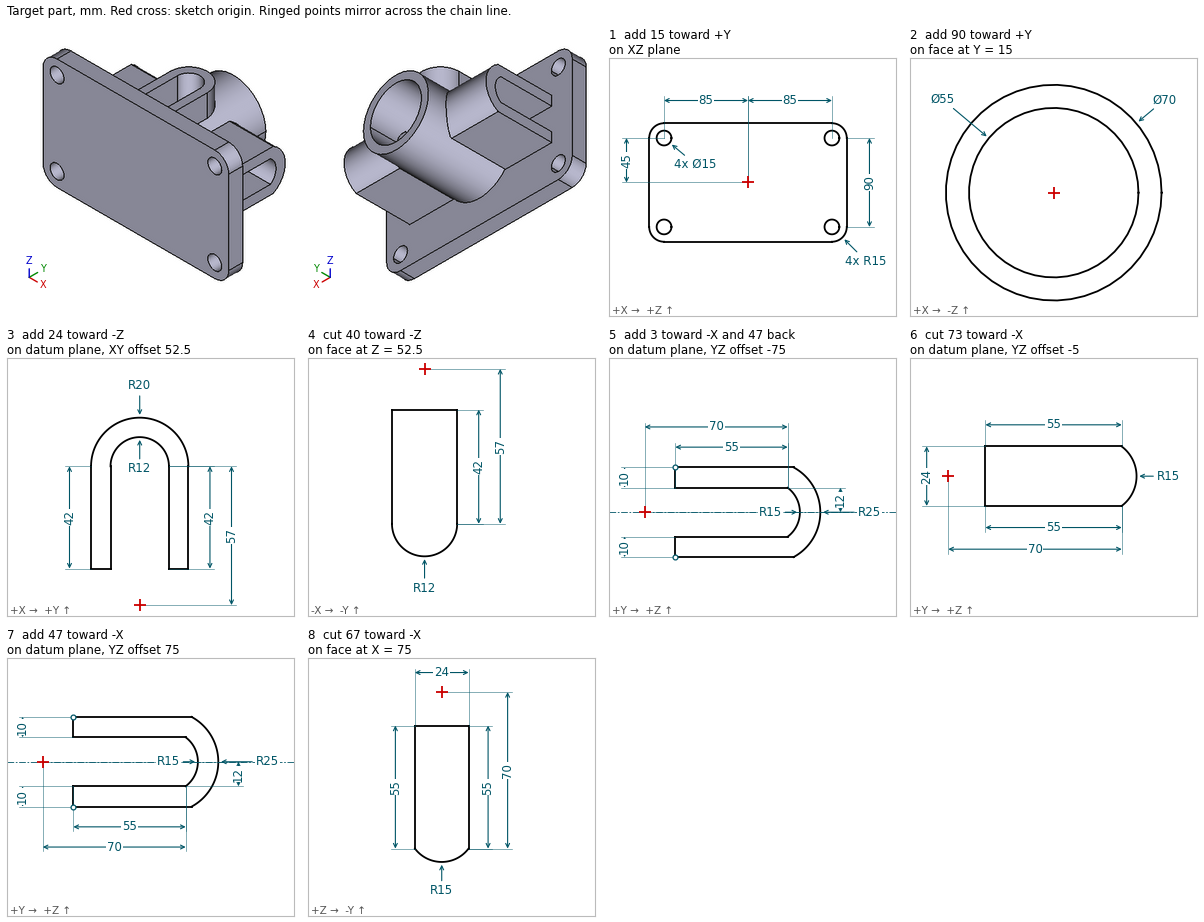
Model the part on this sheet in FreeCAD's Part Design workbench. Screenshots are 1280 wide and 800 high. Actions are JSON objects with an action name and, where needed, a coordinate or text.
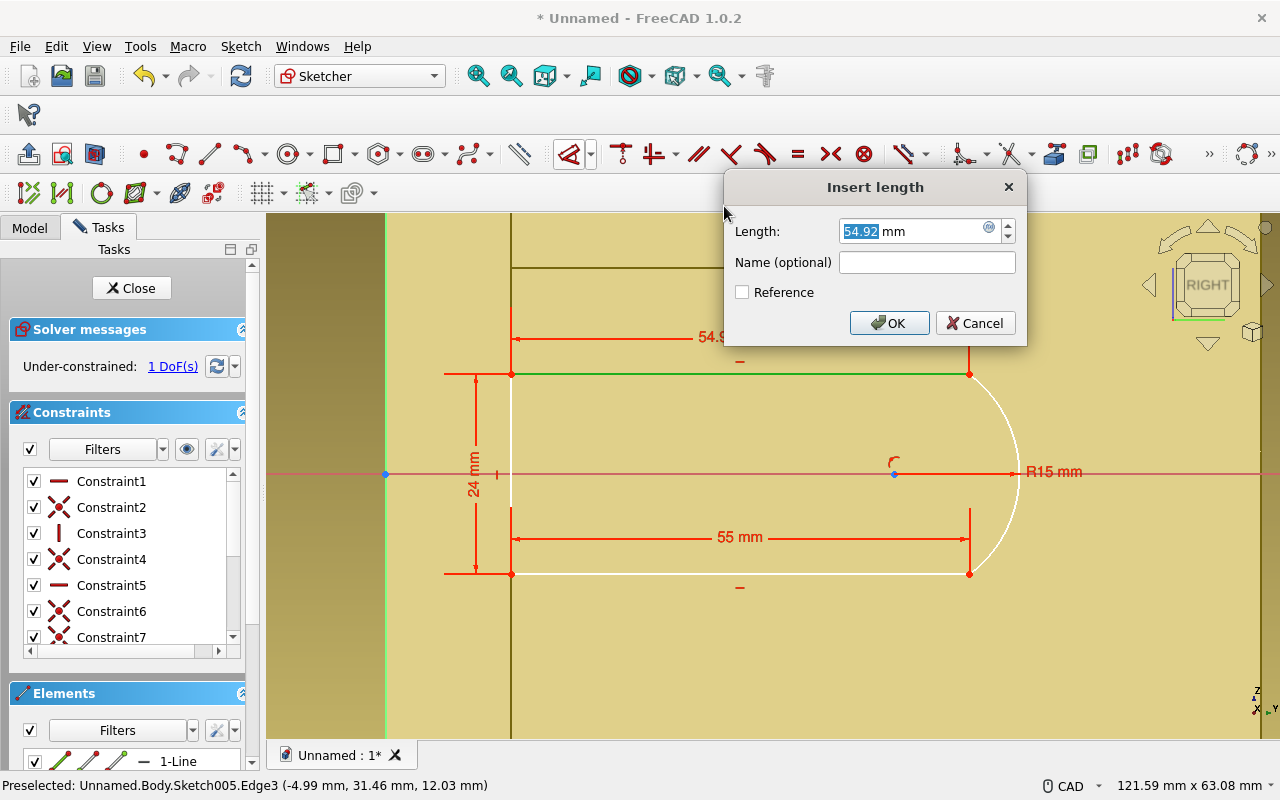
{"action": "type", "text": "55"}
{"action": "key", "text": "Return"}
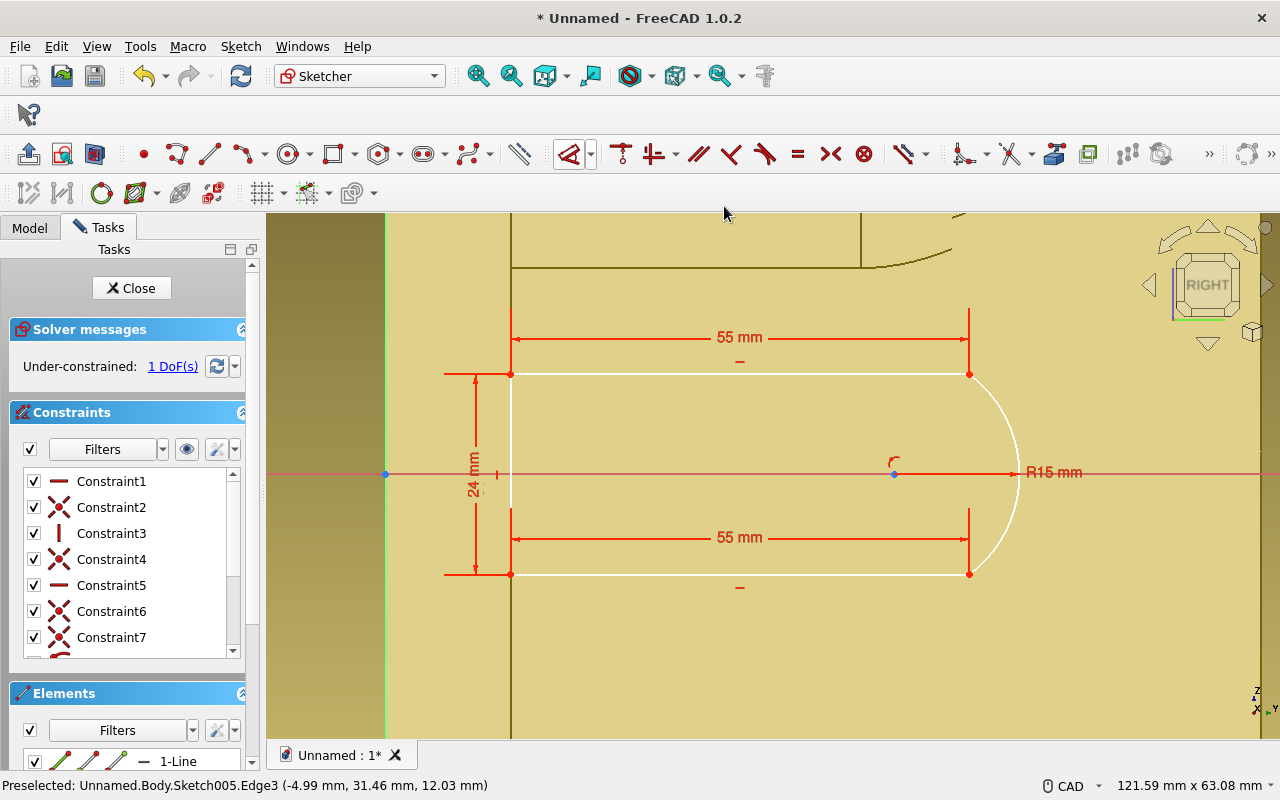
{"action": "left_click", "coordinate": [969, 575]}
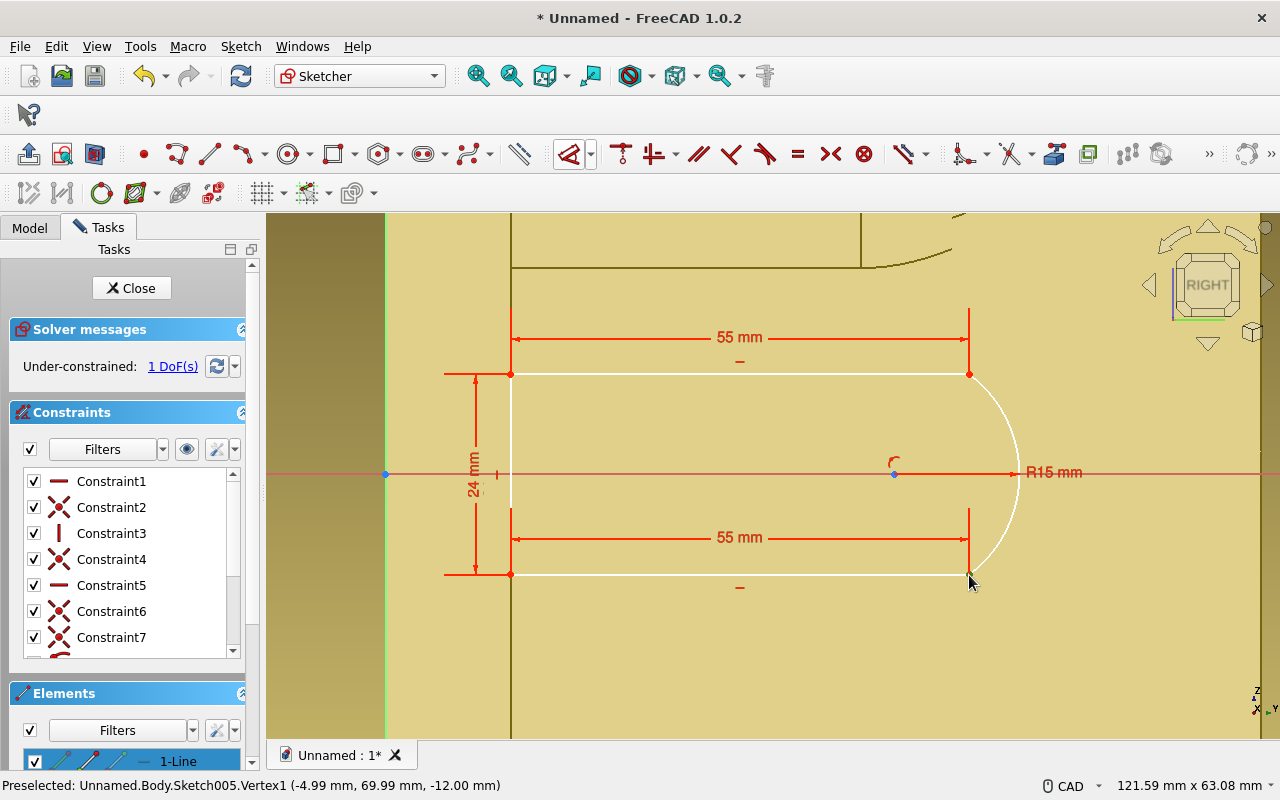
{"action": "key", "text": "l"}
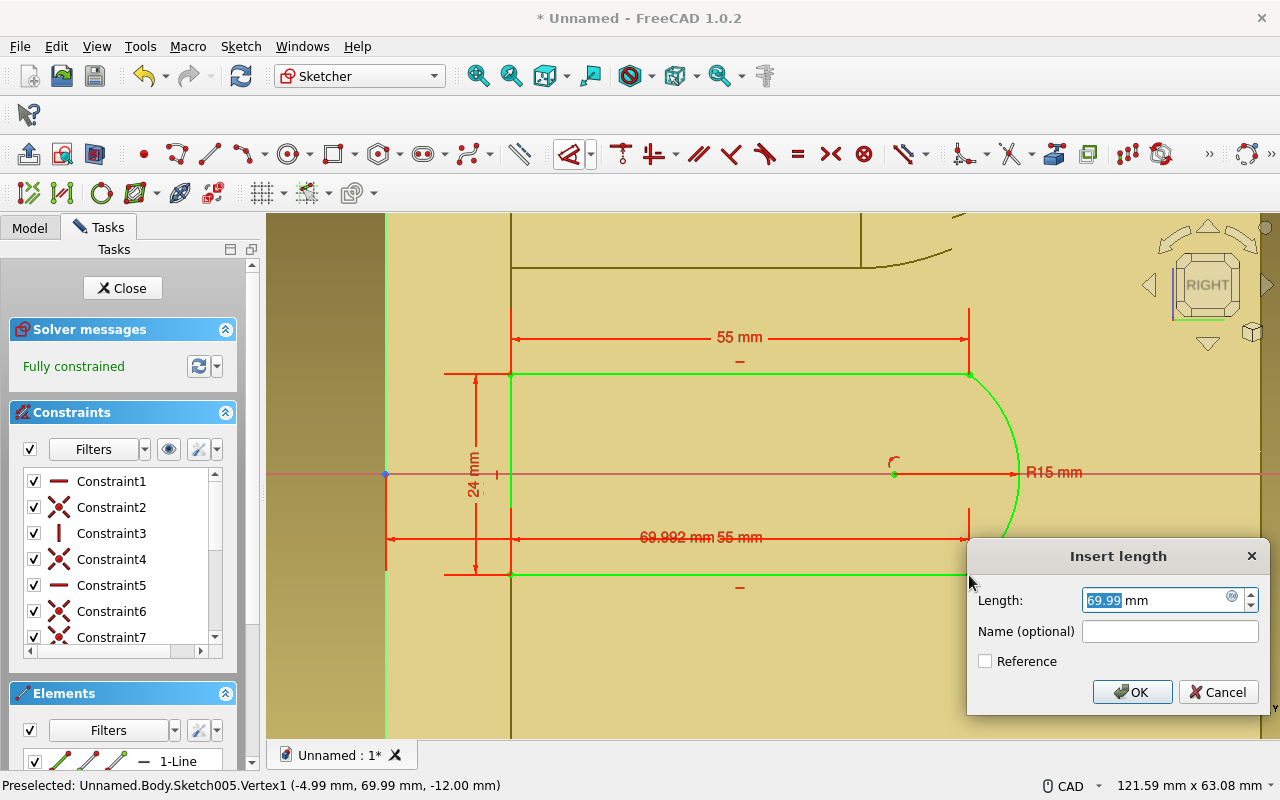
{"action": "type", "text": "70"}
{"action": "key", "text": "Return"}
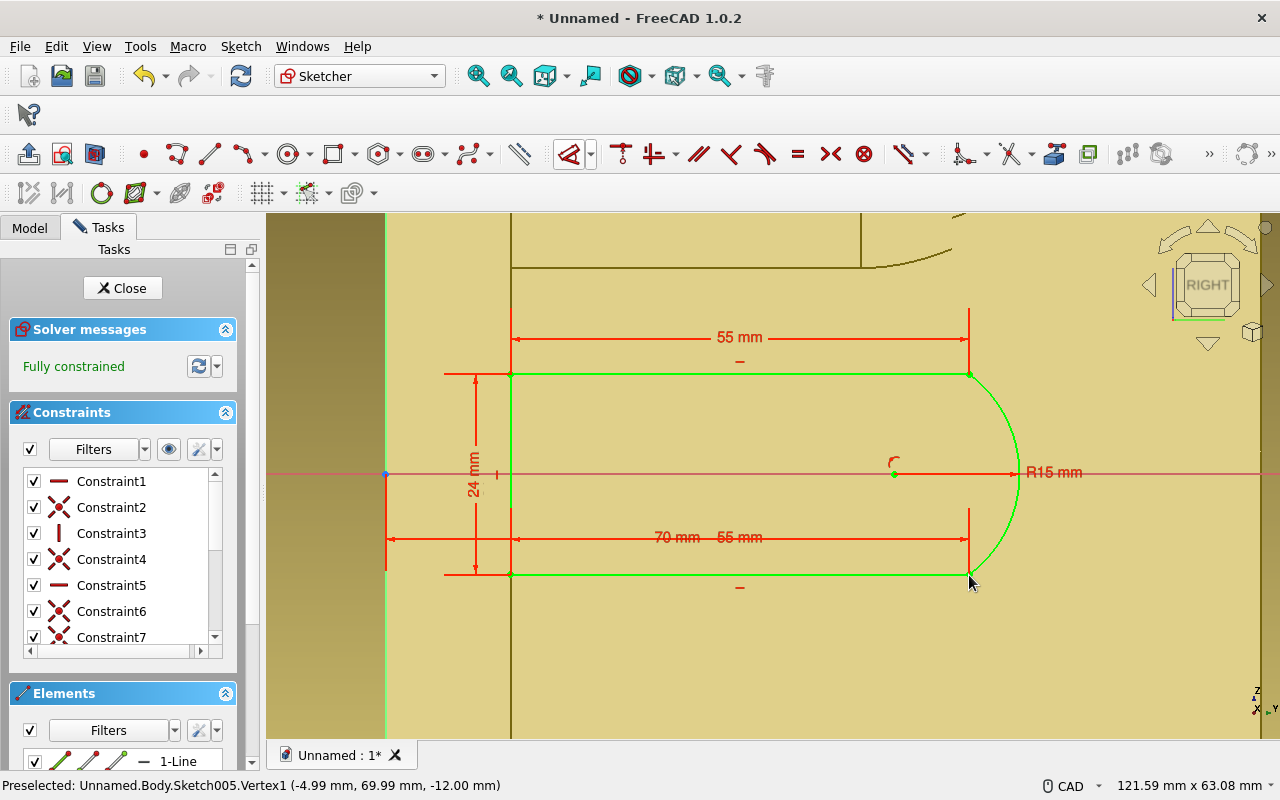
{"action": "left_click", "coordinate": [123, 288]}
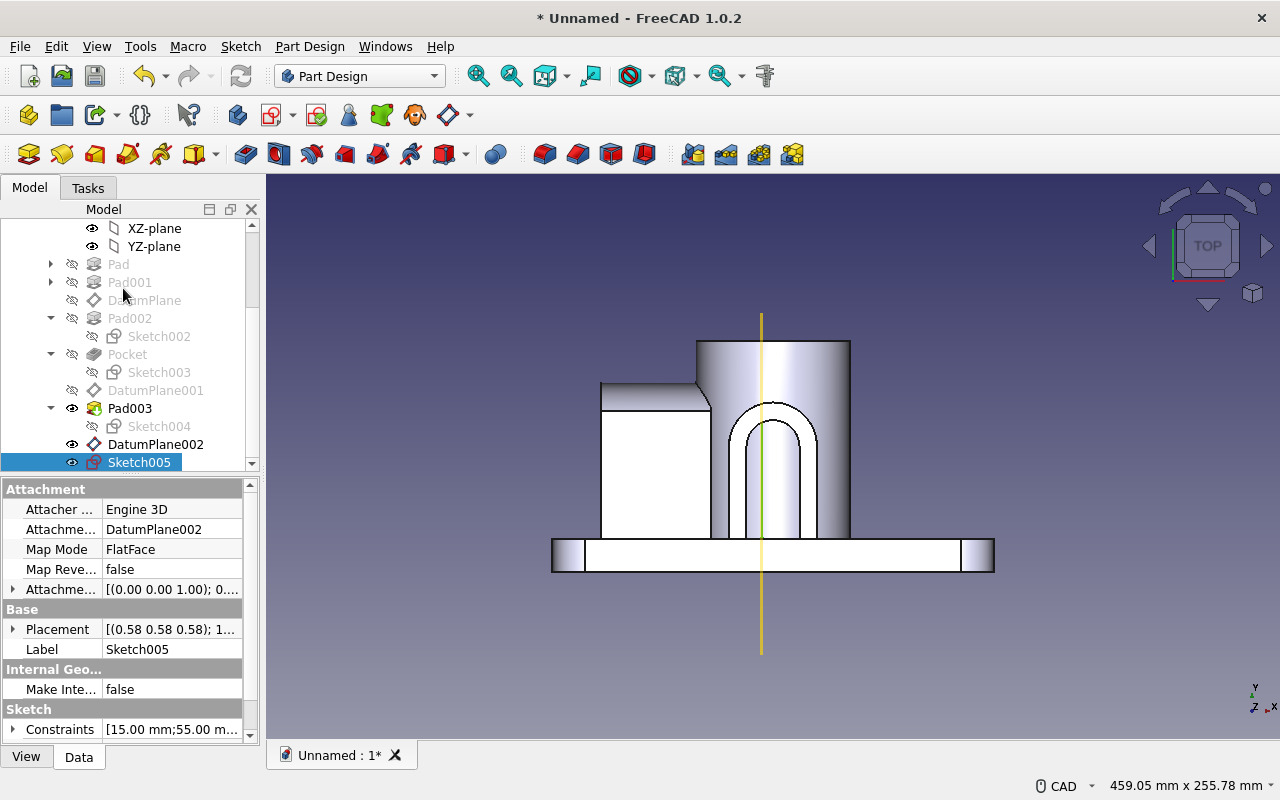
{"action": "left_click", "coordinate": [246, 154]}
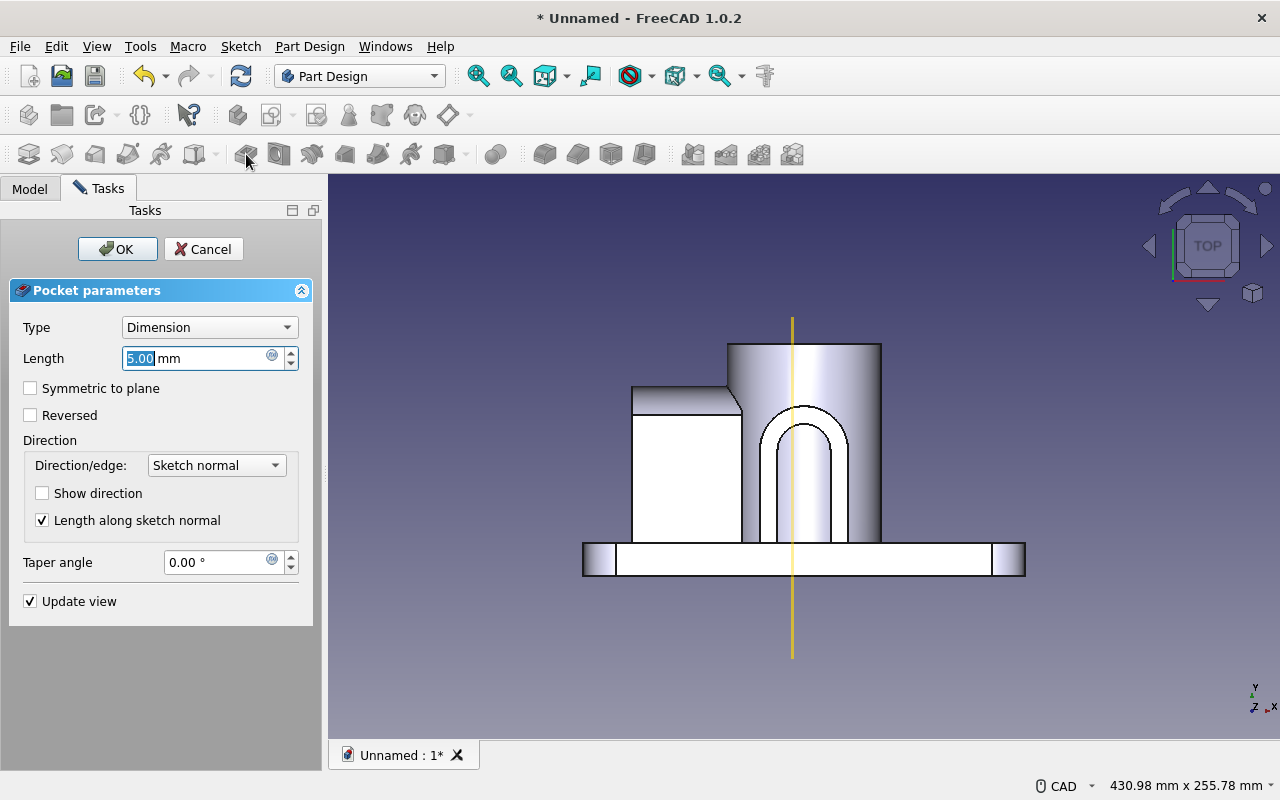
{"action": "type", "text": "73"}
{"action": "key", "text": "Tab"}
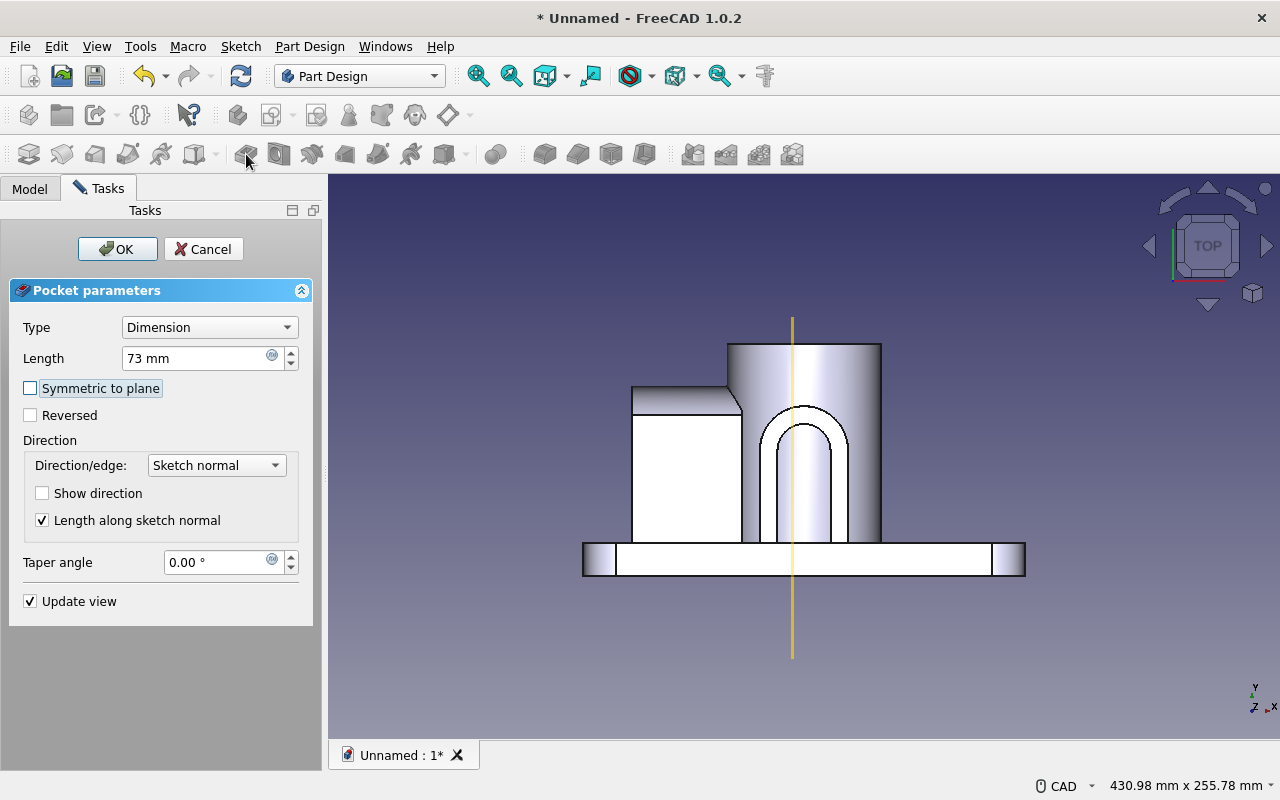
{"action": "left_click", "coordinate": [118, 249]}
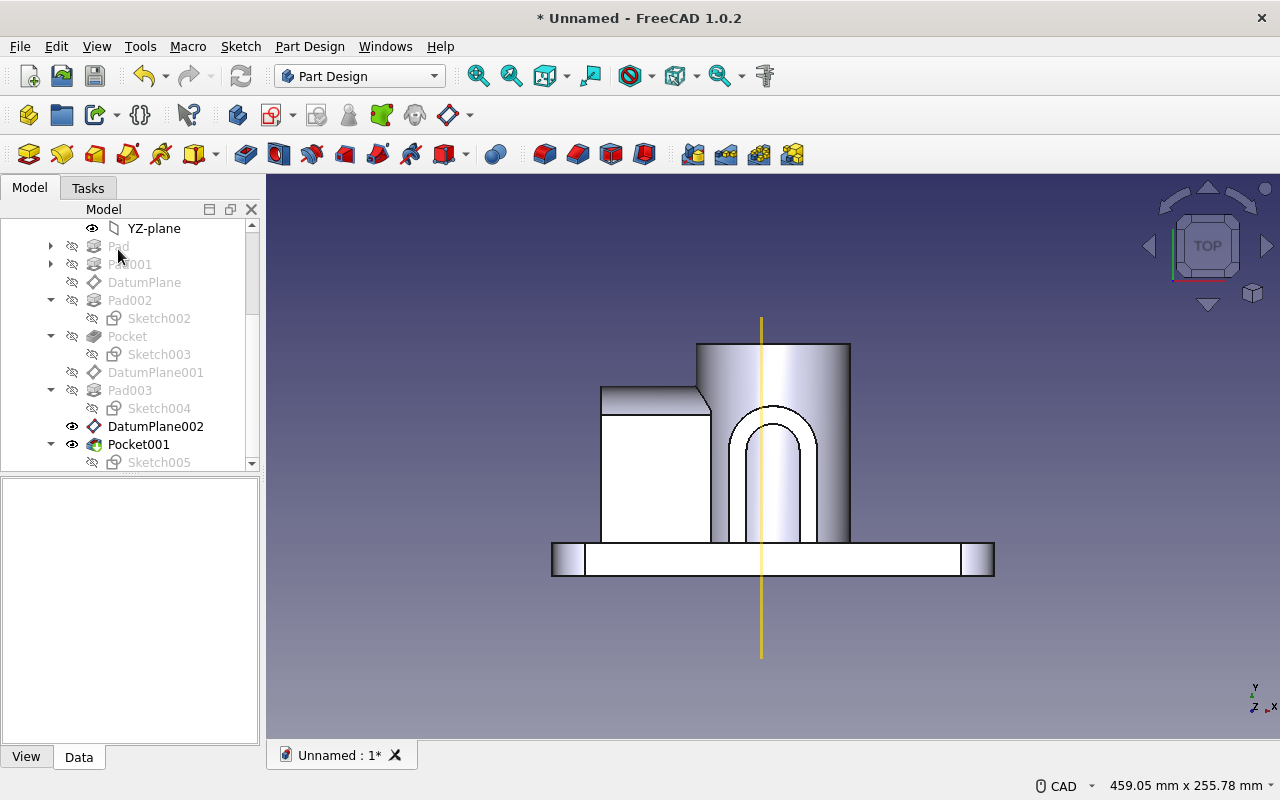
{"action": "left_click", "coordinate": [117, 426]}
{"action": "key", "text": "space"}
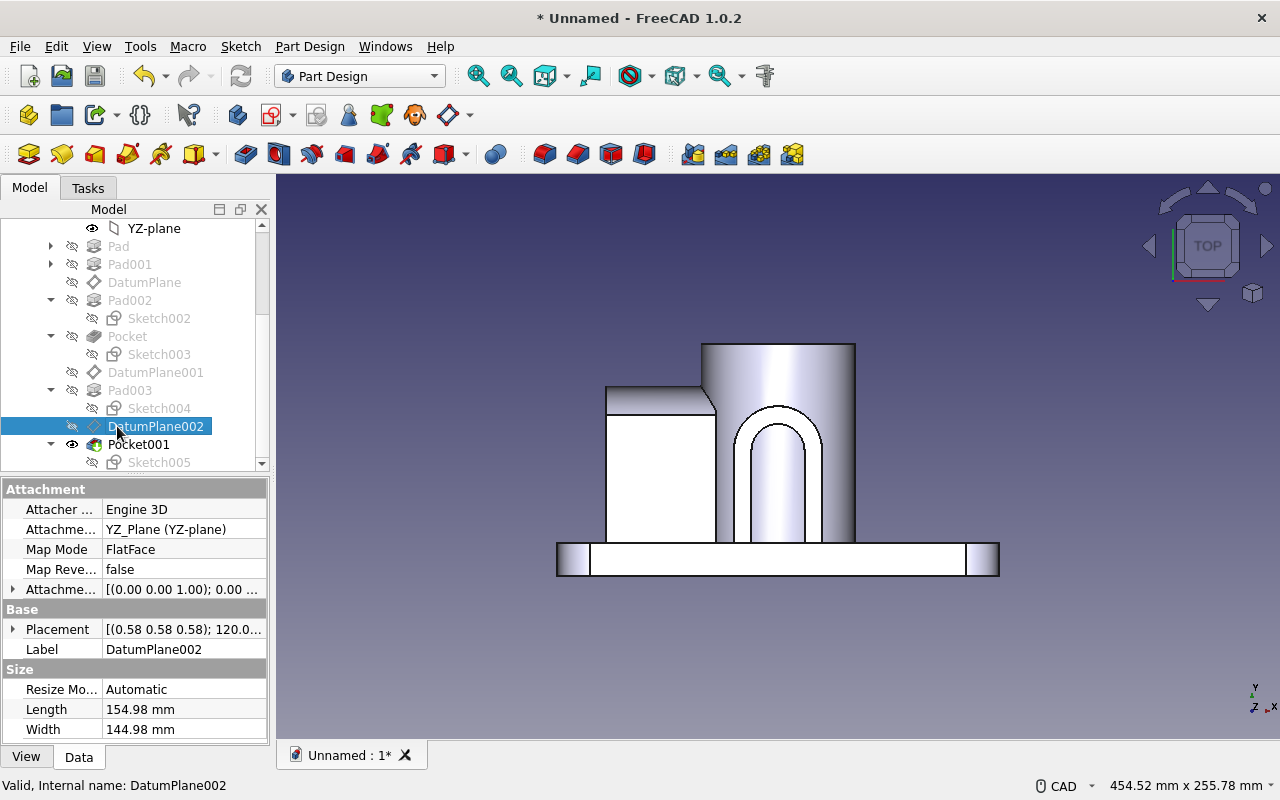
{"action": "key", "text": "v f"}